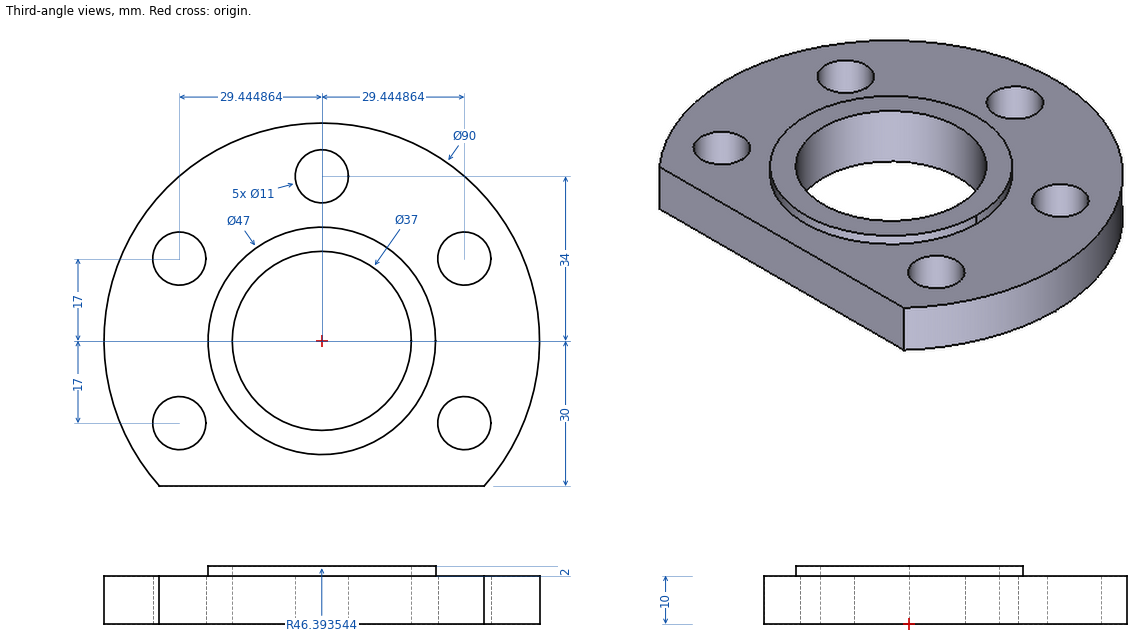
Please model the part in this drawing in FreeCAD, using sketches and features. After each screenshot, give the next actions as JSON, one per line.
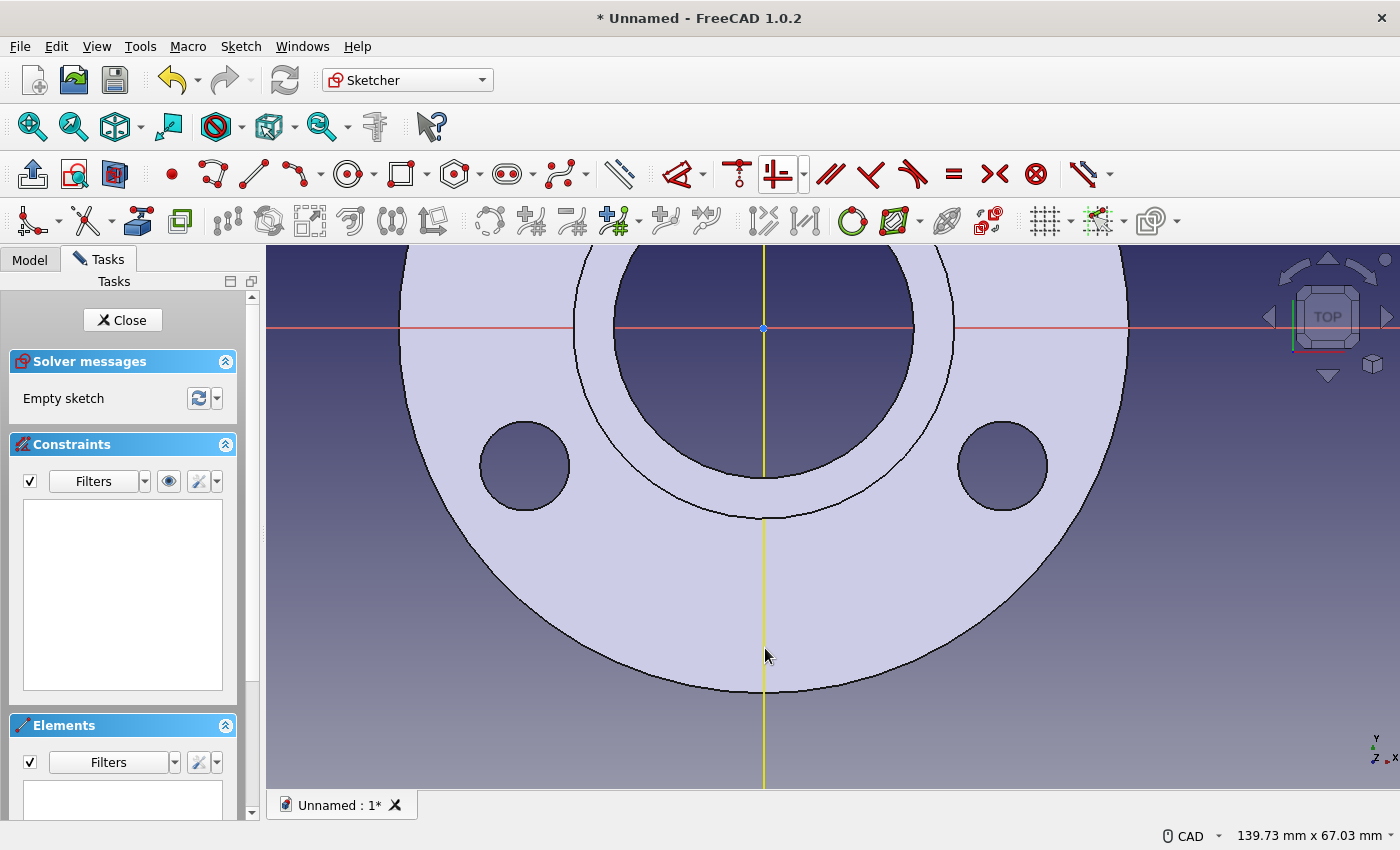
{"action": "left_click", "coordinate": [254, 174]}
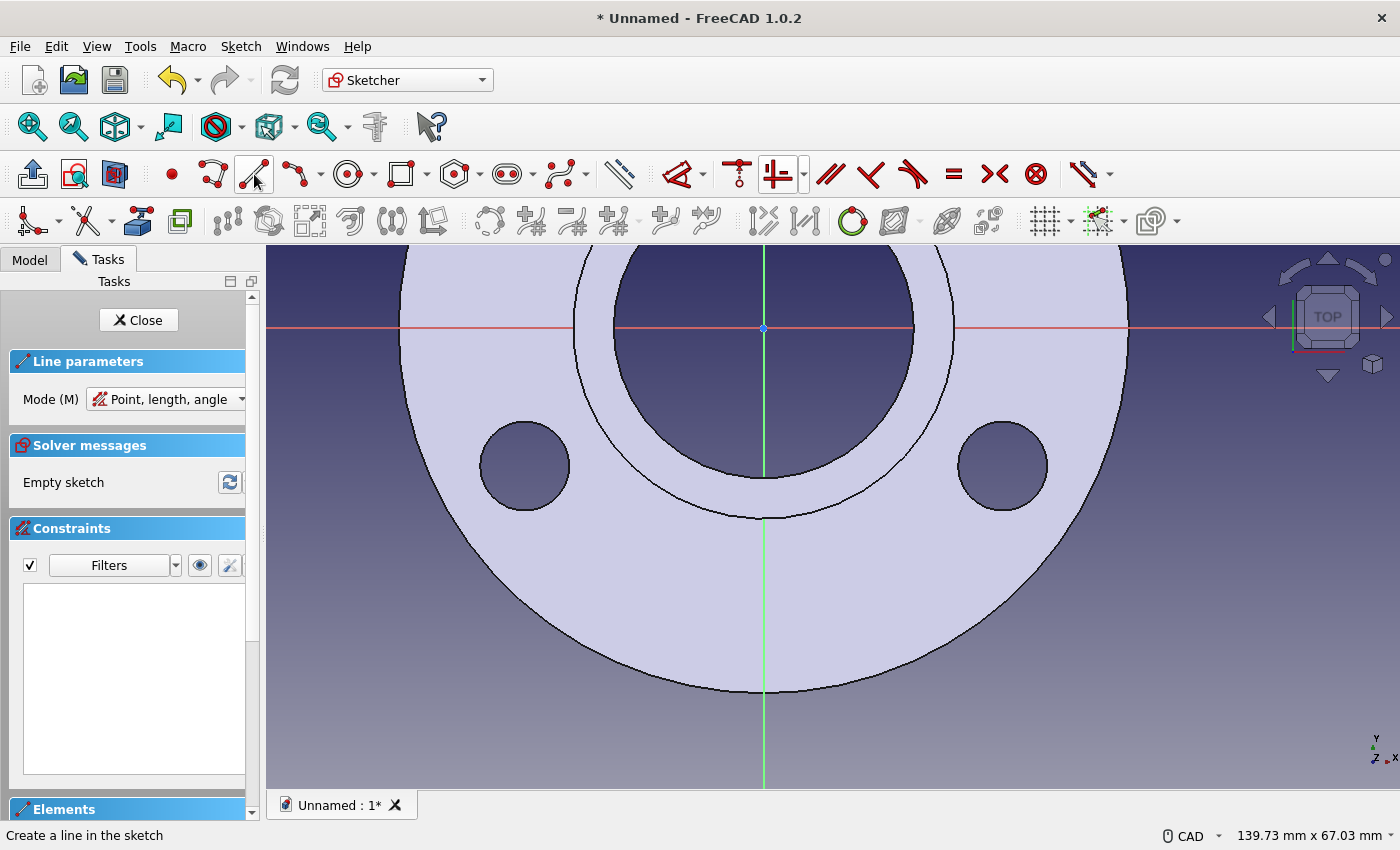
{"action": "left_click", "coordinate": [1051, 572]}
{"action": "left_click", "coordinate": [477, 572]}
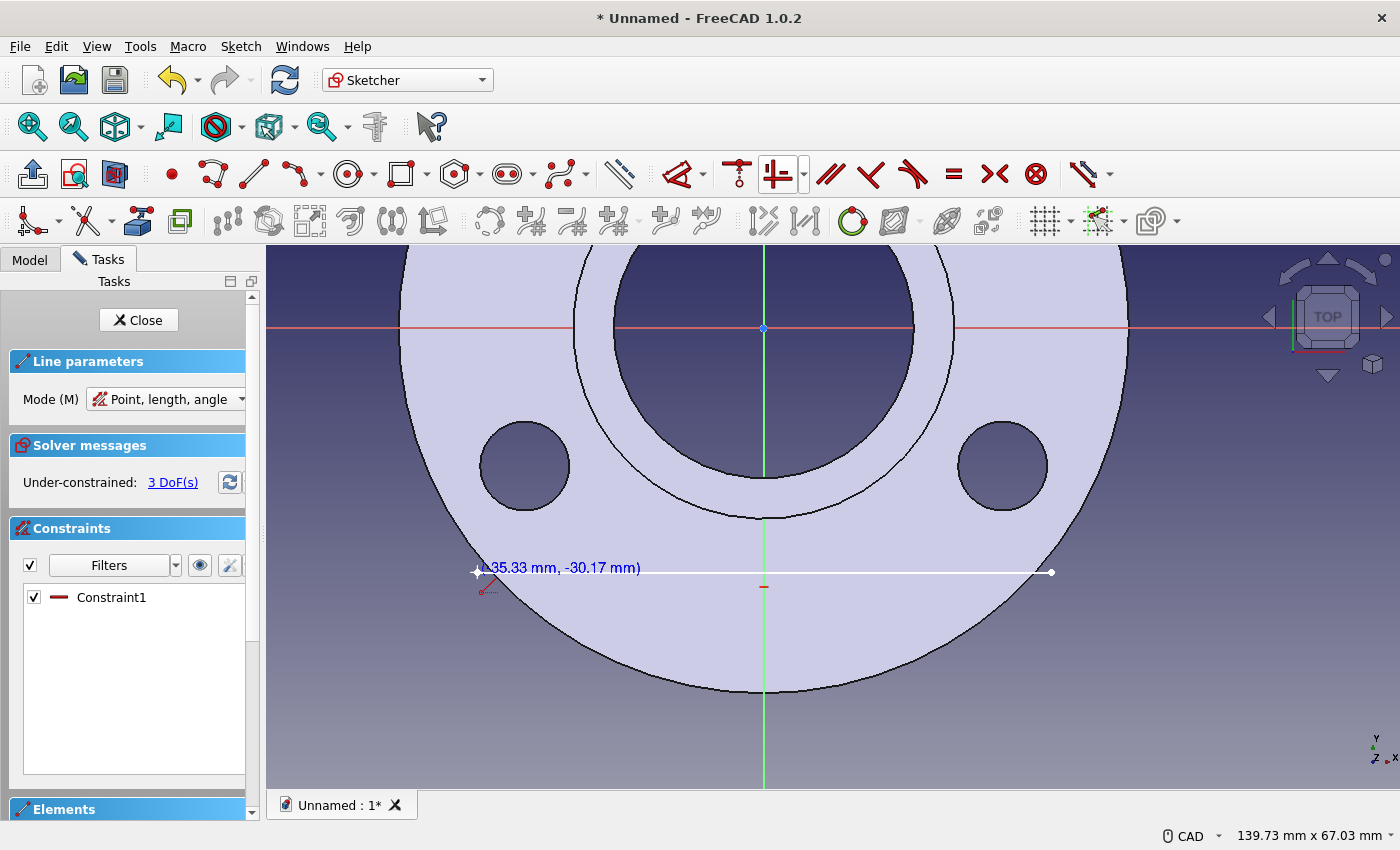
{"action": "key", "text": "g 3 a"}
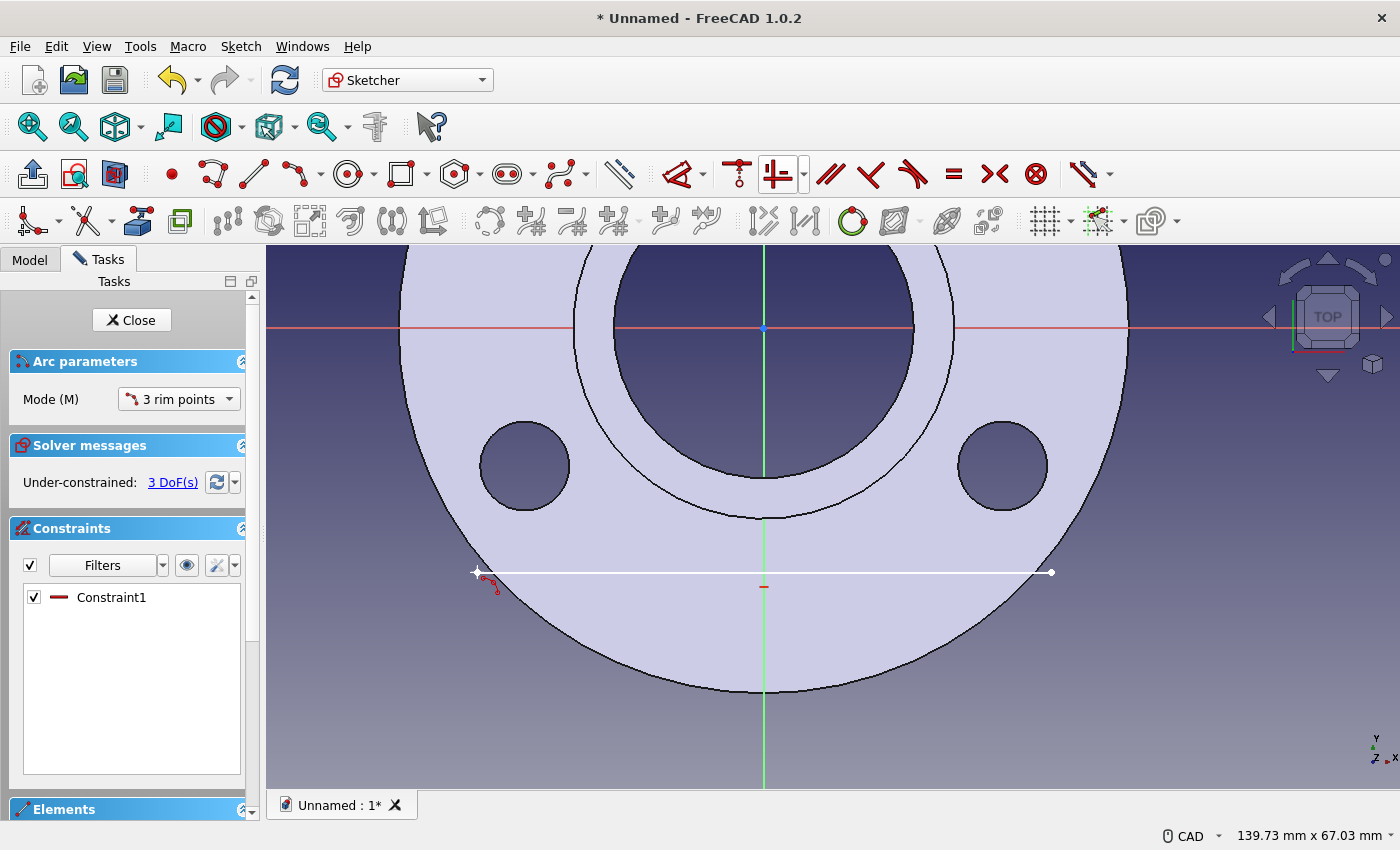
{"action": "left_click", "coordinate": [477, 573]}
{"action": "left_click", "coordinate": [1051, 573]}
{"action": "left_click", "coordinate": [699, 699]}
{"action": "key", "text": "Escape"}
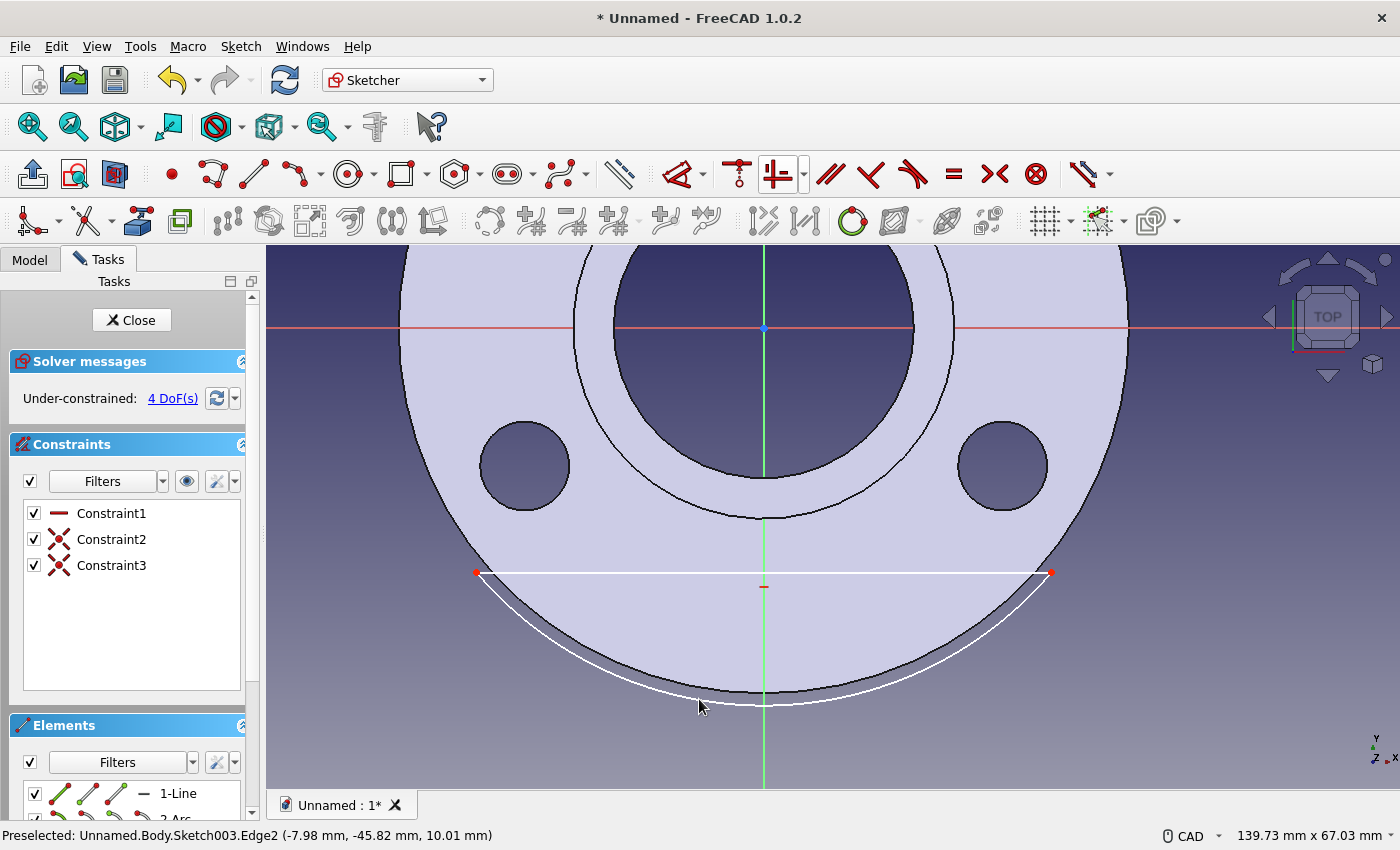
{"action": "left_click_drag", "start_coordinate": [754, 318], "coordinate": [774, 339]}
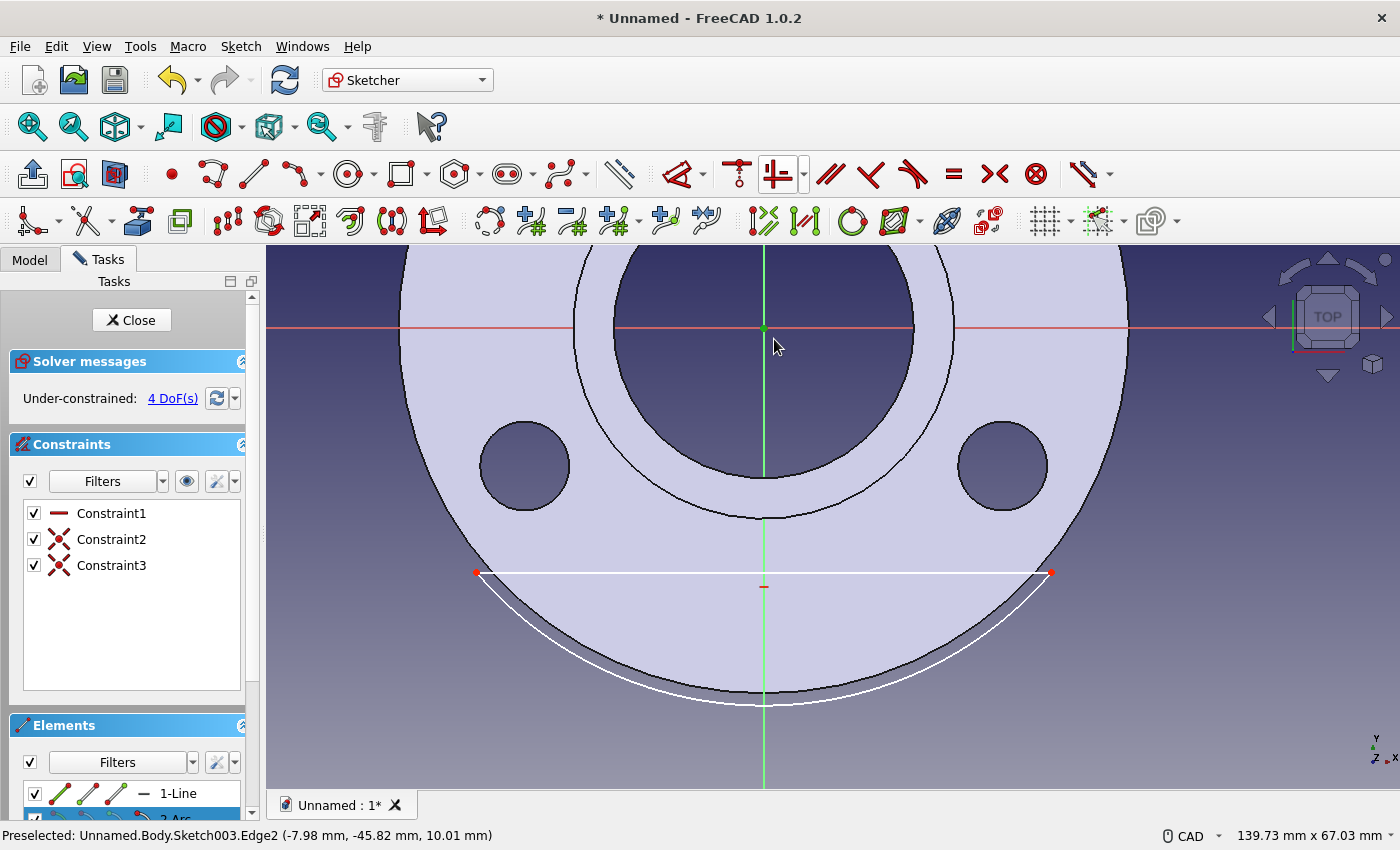
{"action": "left_click", "coordinate": [737, 174]}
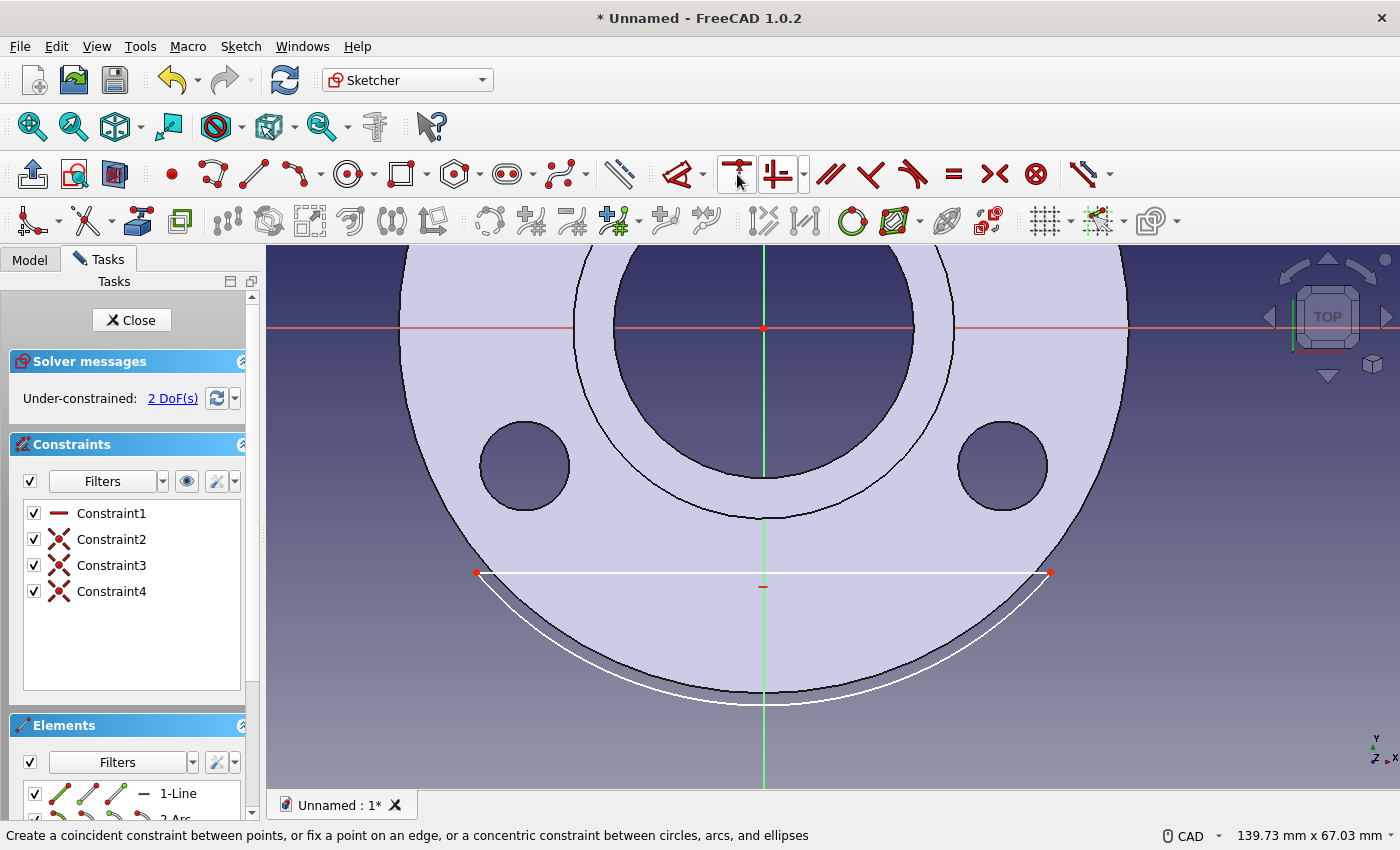
{"action": "left_click", "coordinate": [676, 174]}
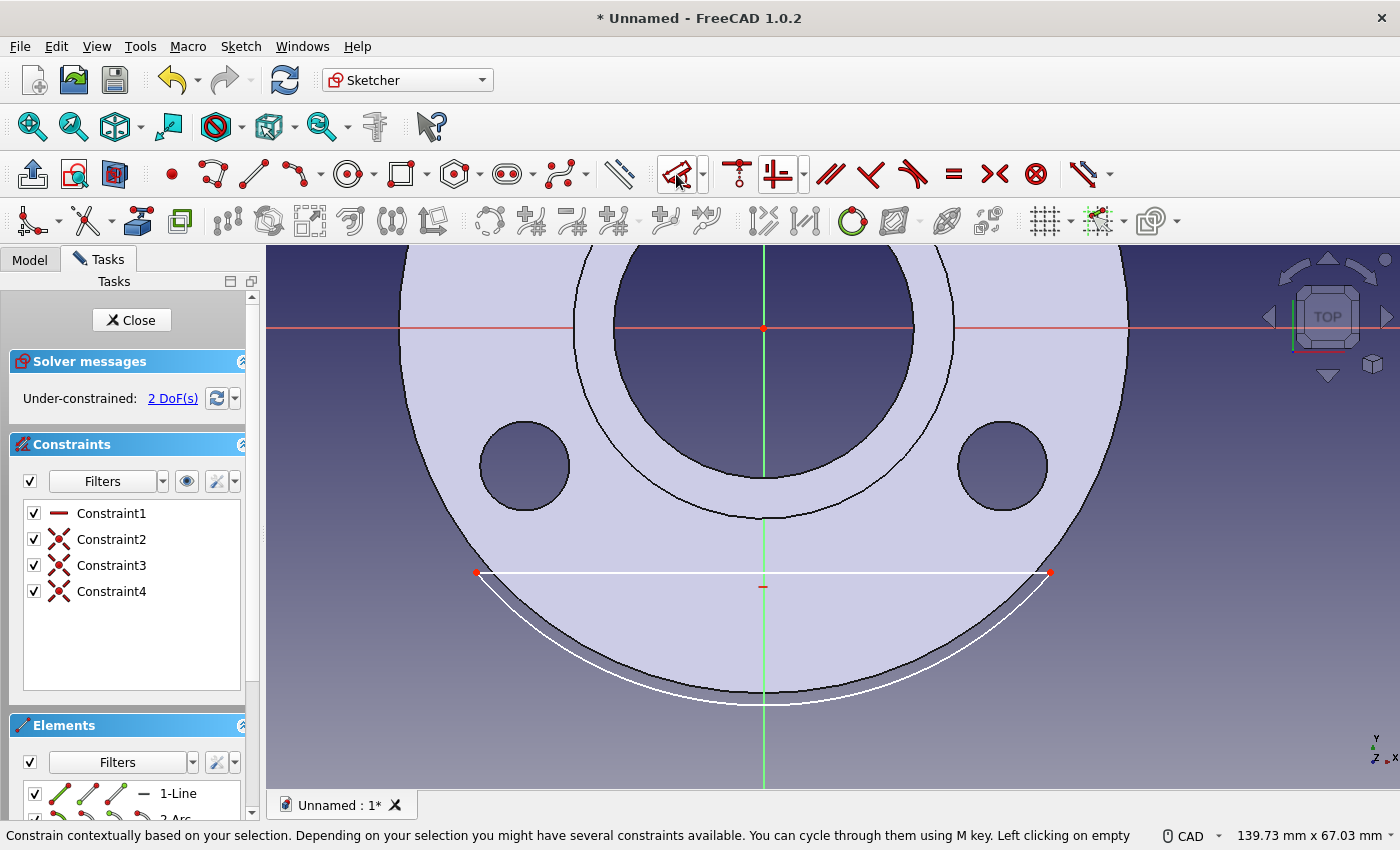
{"action": "left_click", "coordinate": [636, 683]}
{"action": "left_click", "coordinate": [625, 713]}